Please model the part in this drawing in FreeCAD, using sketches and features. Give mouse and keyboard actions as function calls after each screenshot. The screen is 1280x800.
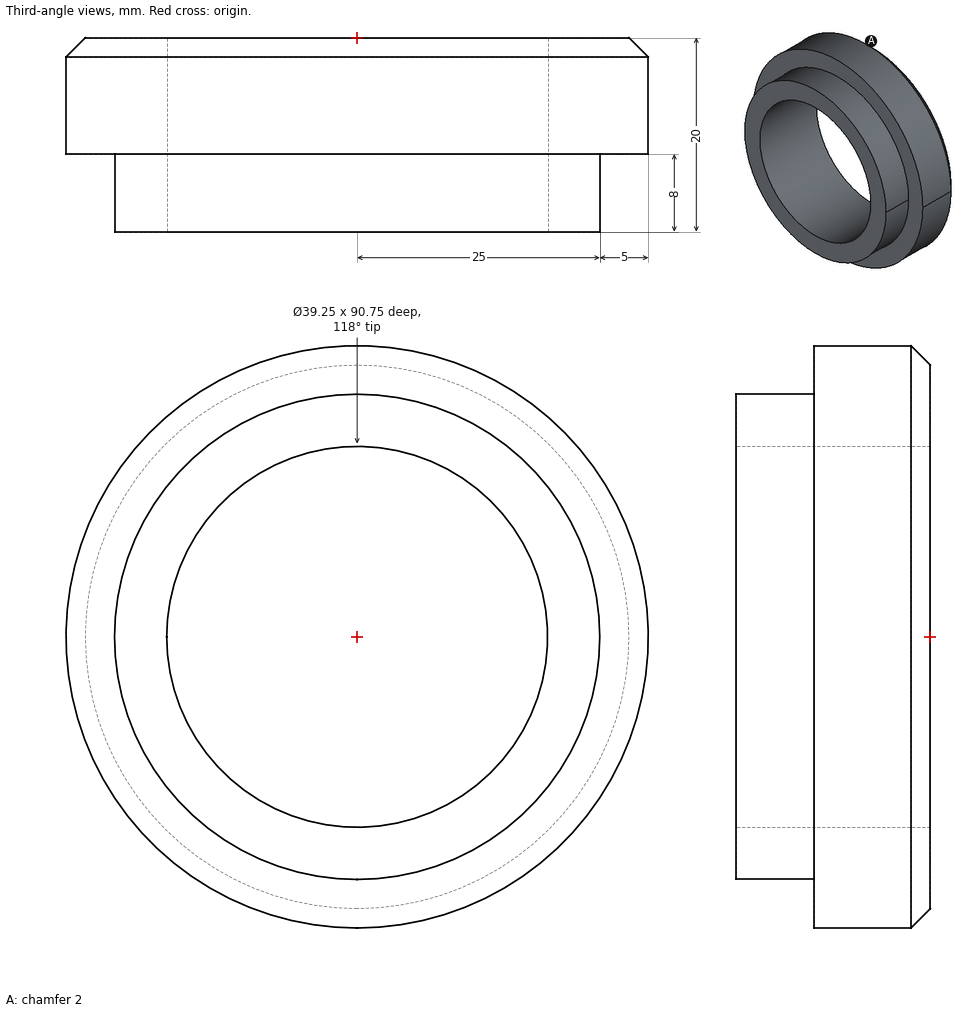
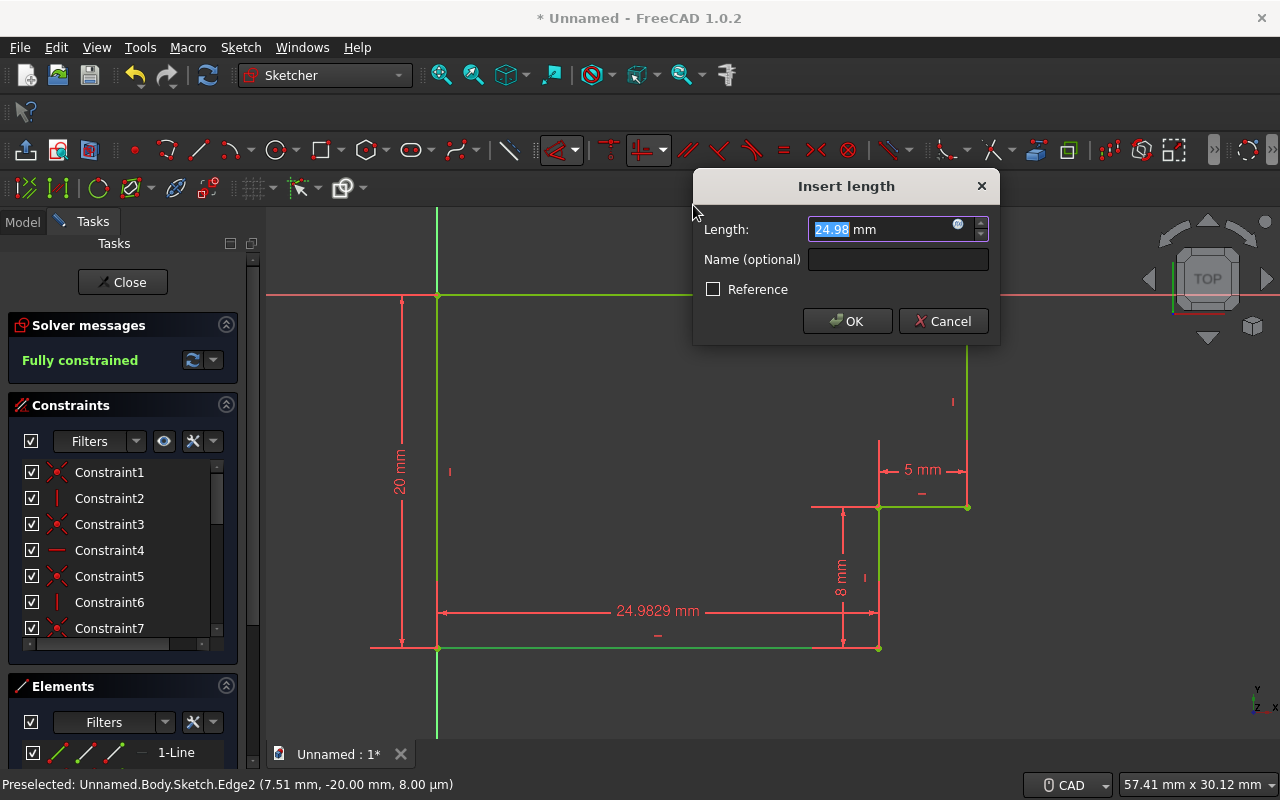
text(25)
key(Return)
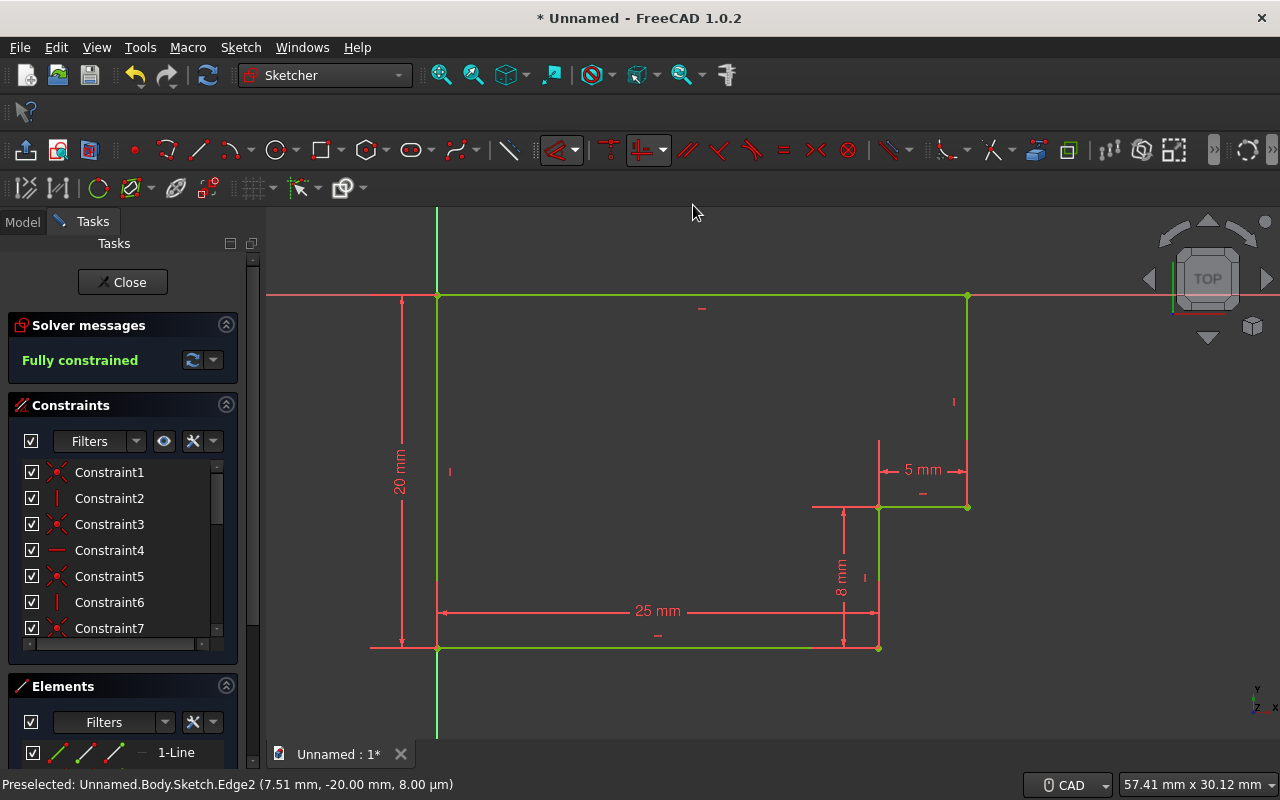
click(123, 282)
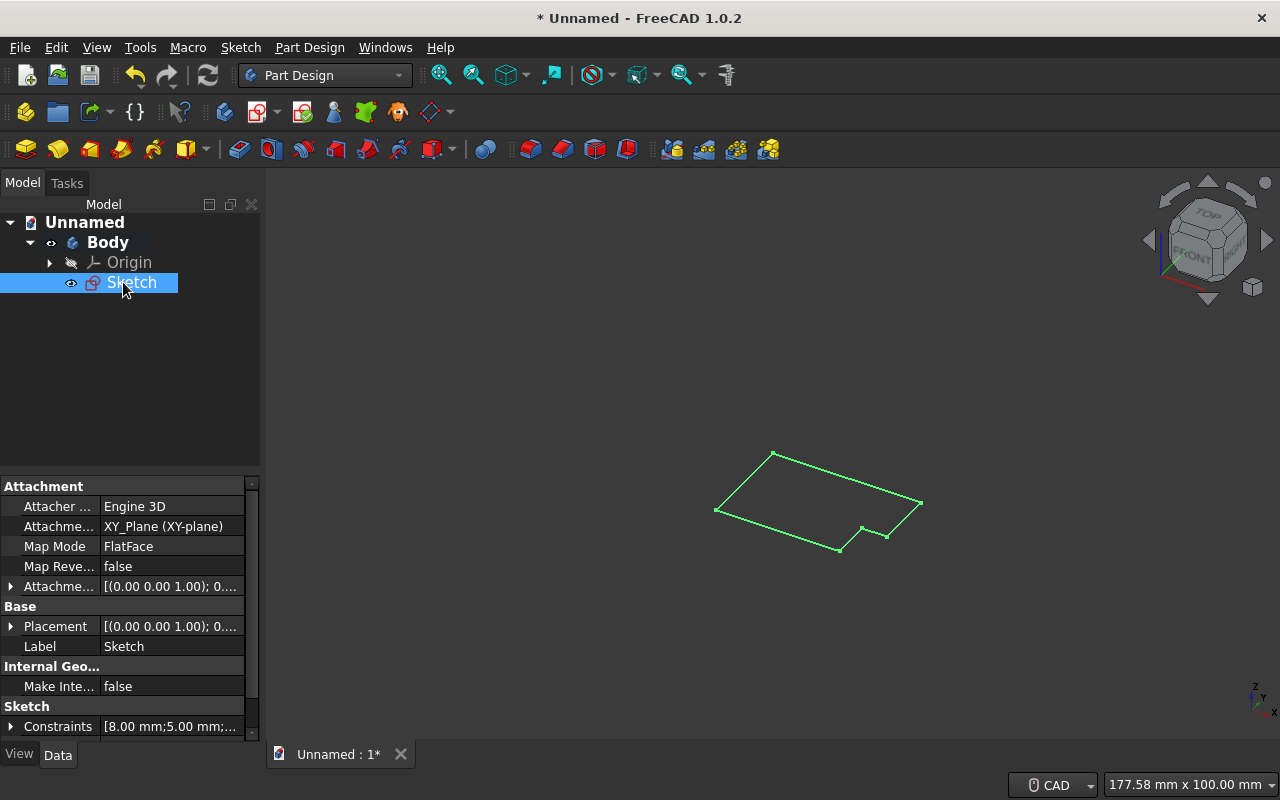
click(58, 150)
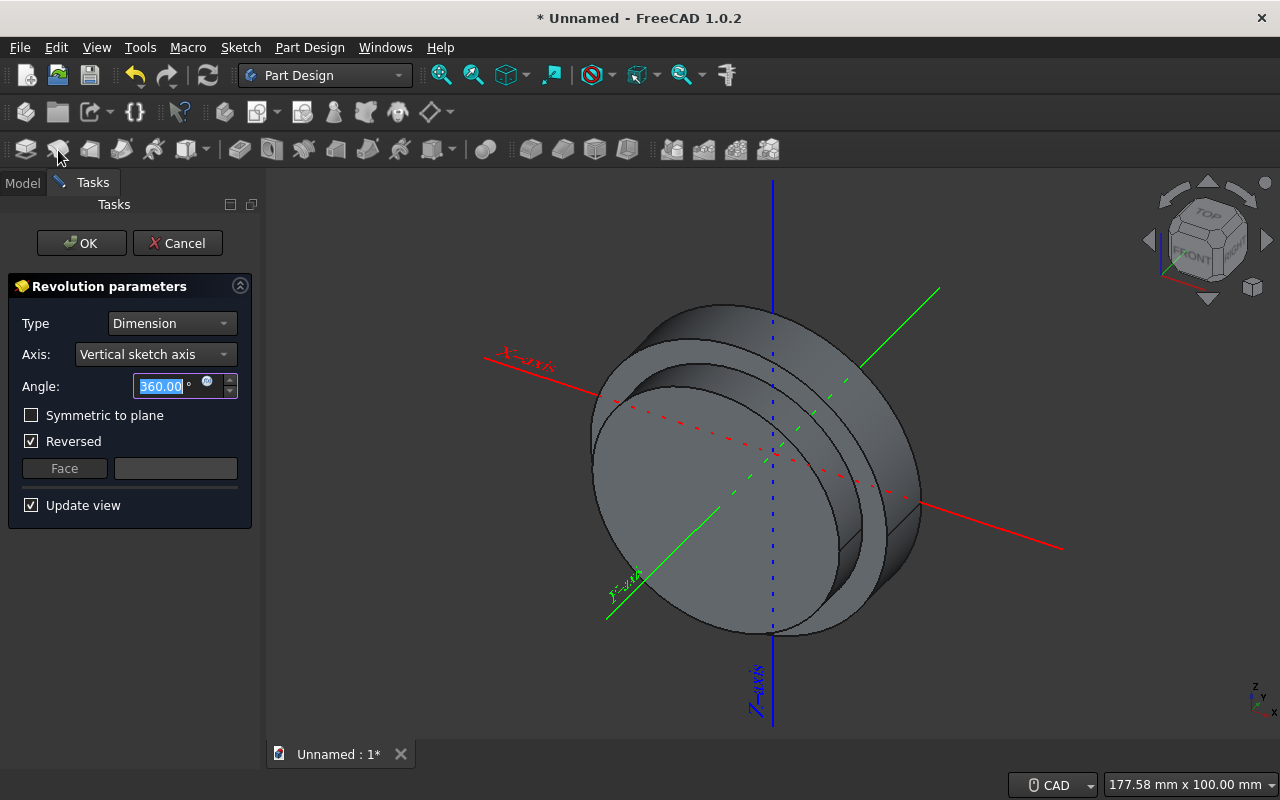
click(82, 243)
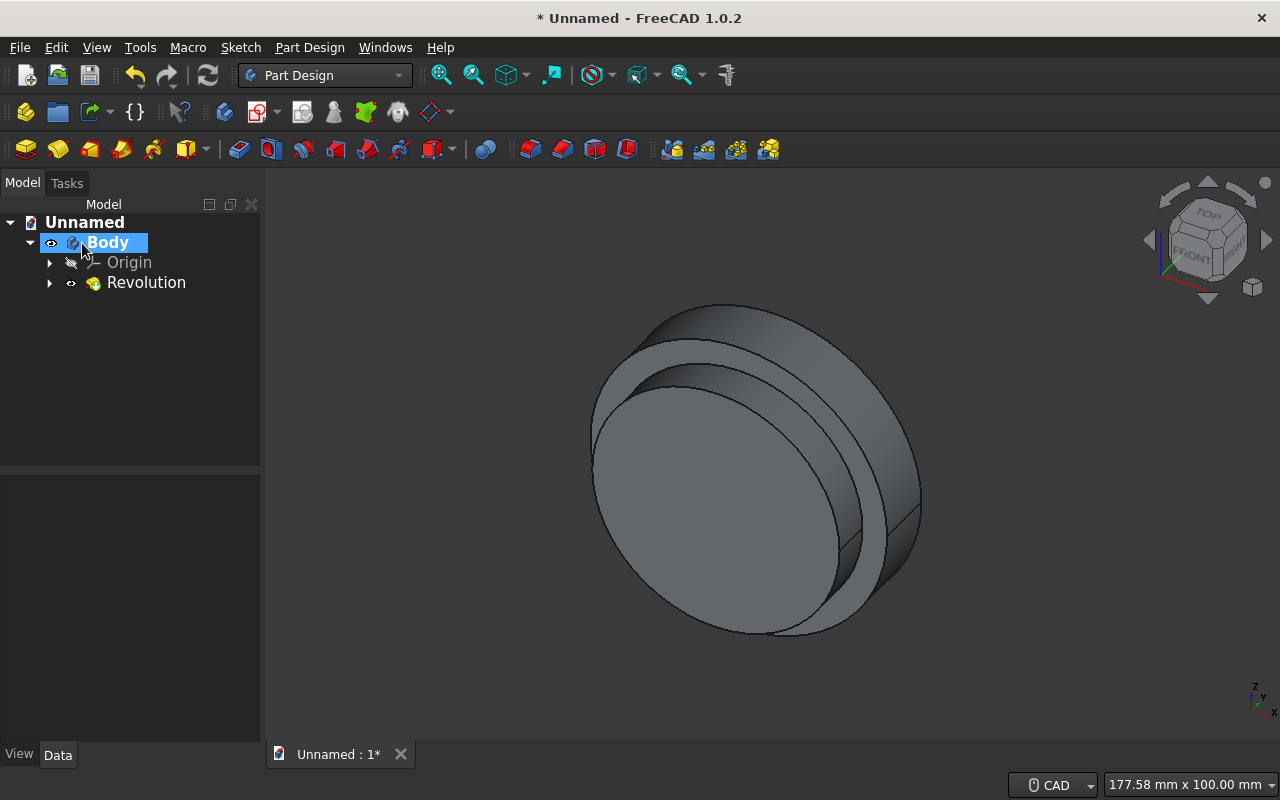
click(258, 112)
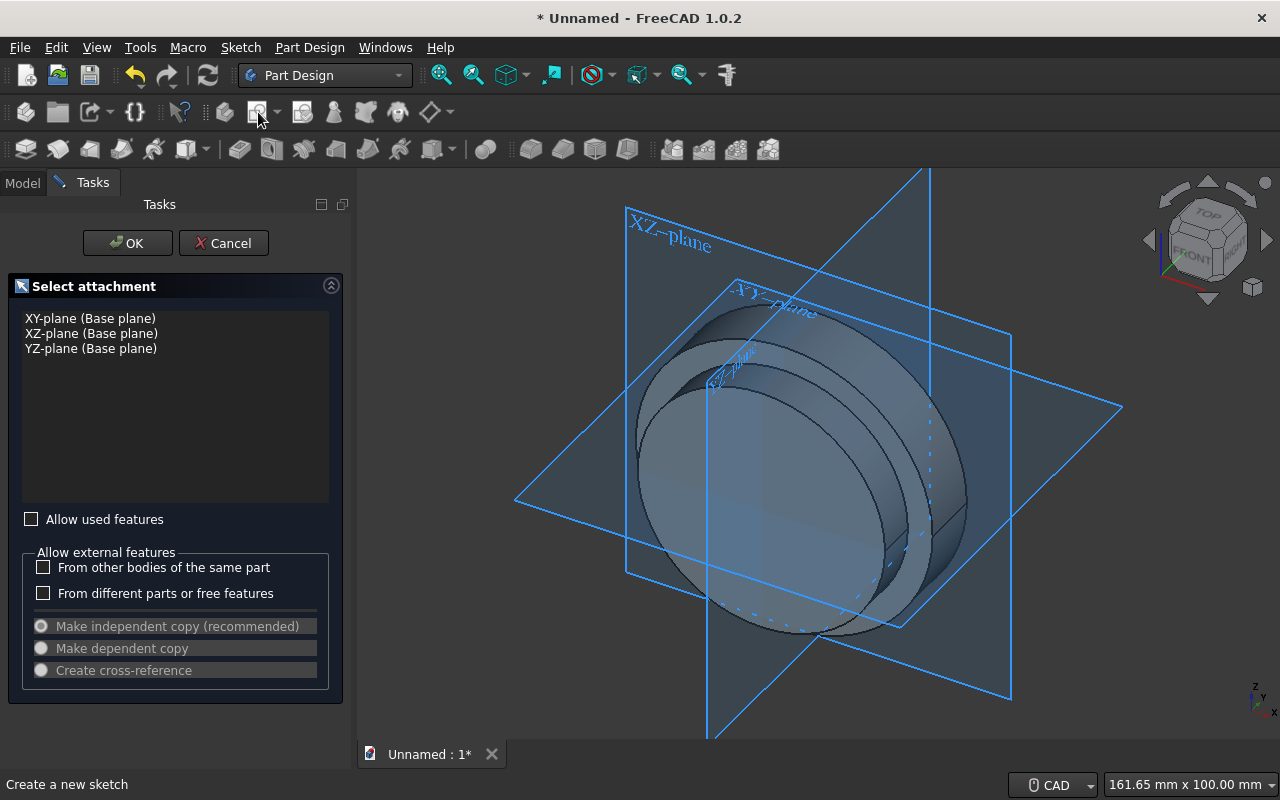
click(82, 334)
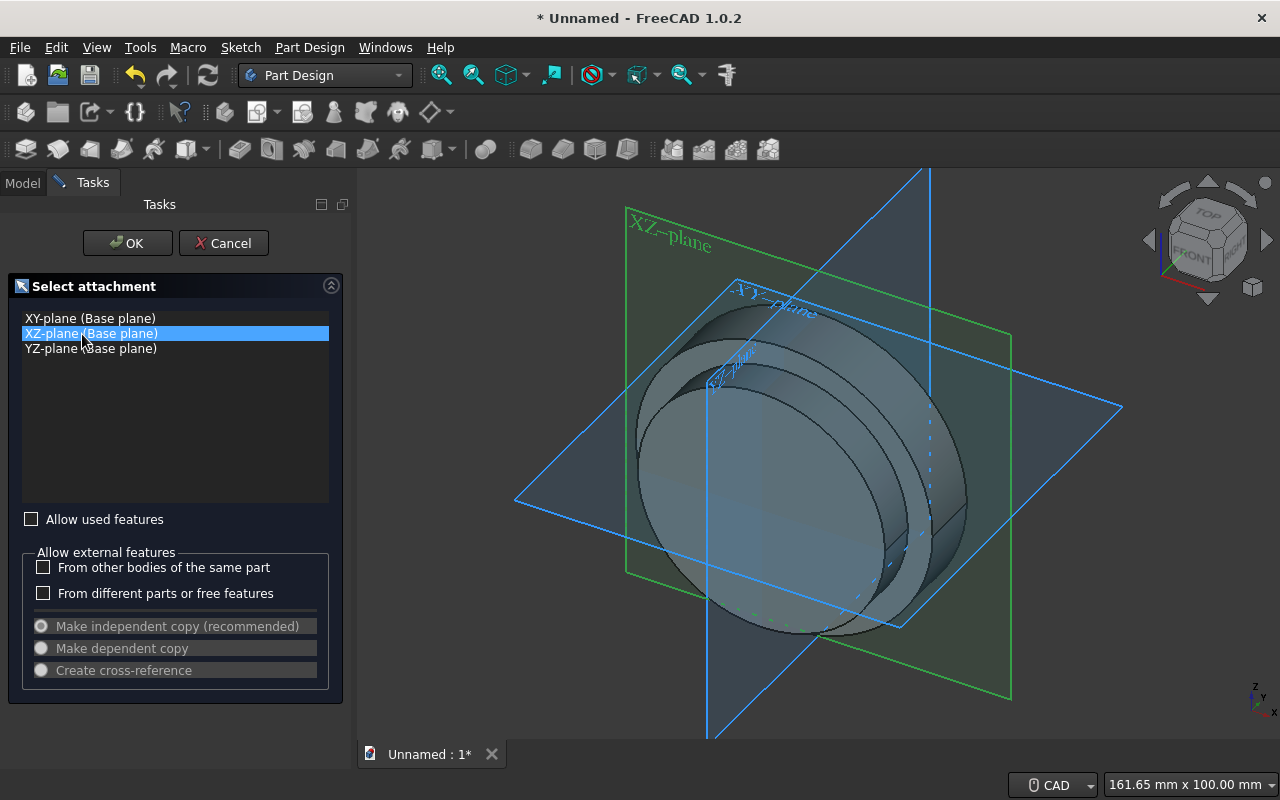
click(128, 243)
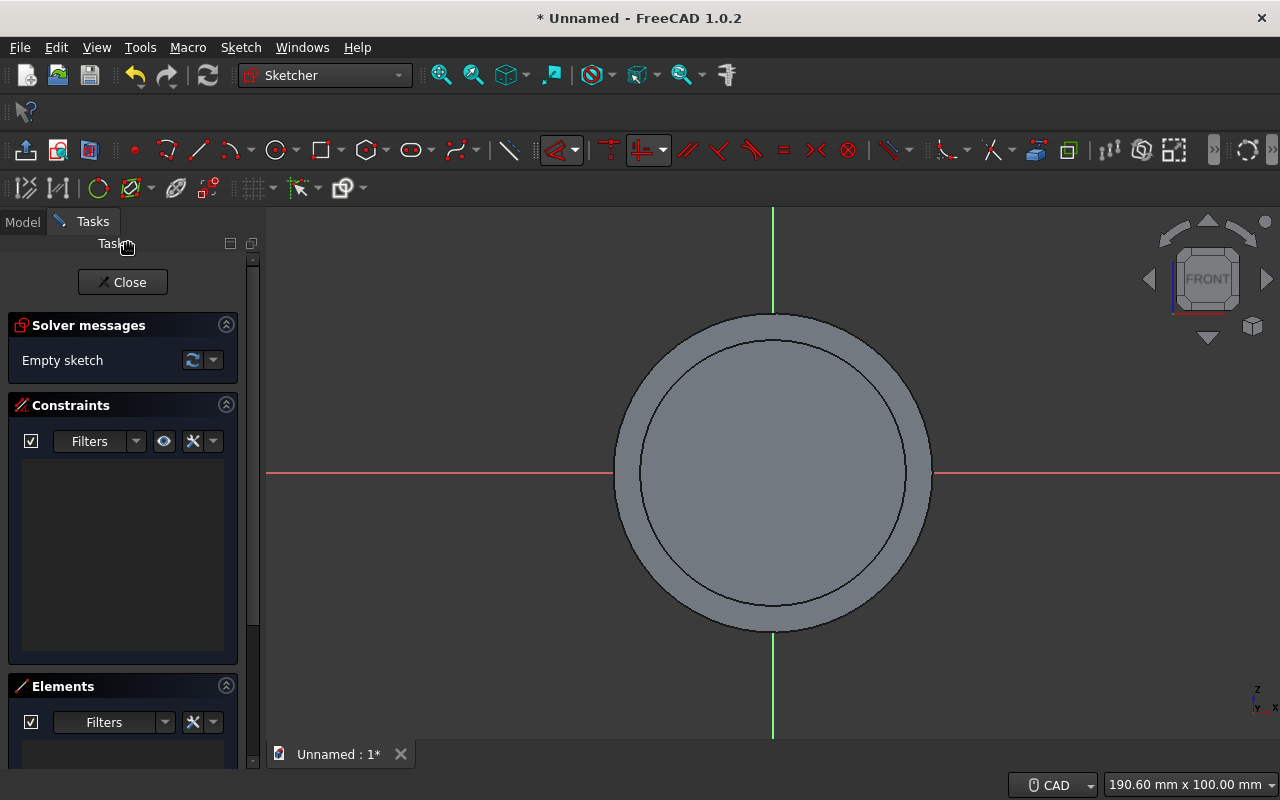
click(90, 150)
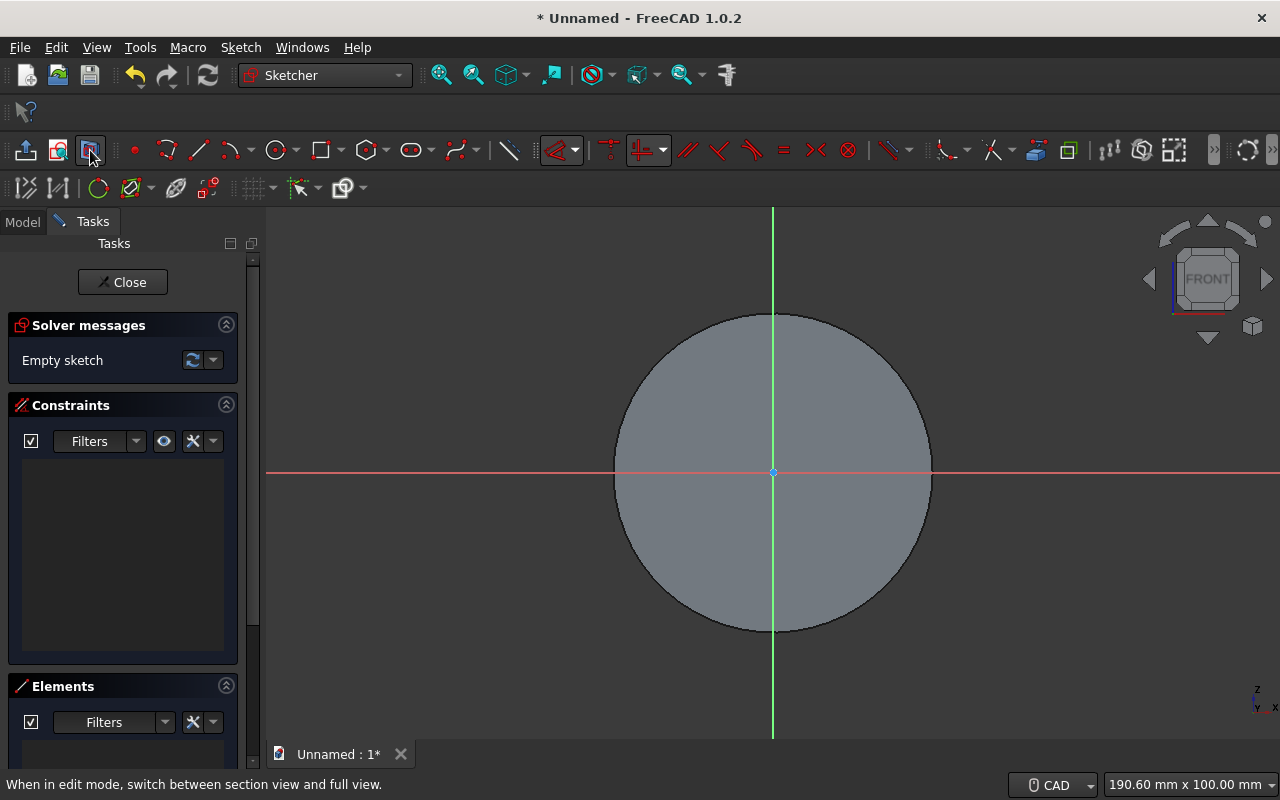
scroll(912, 473, up, 2)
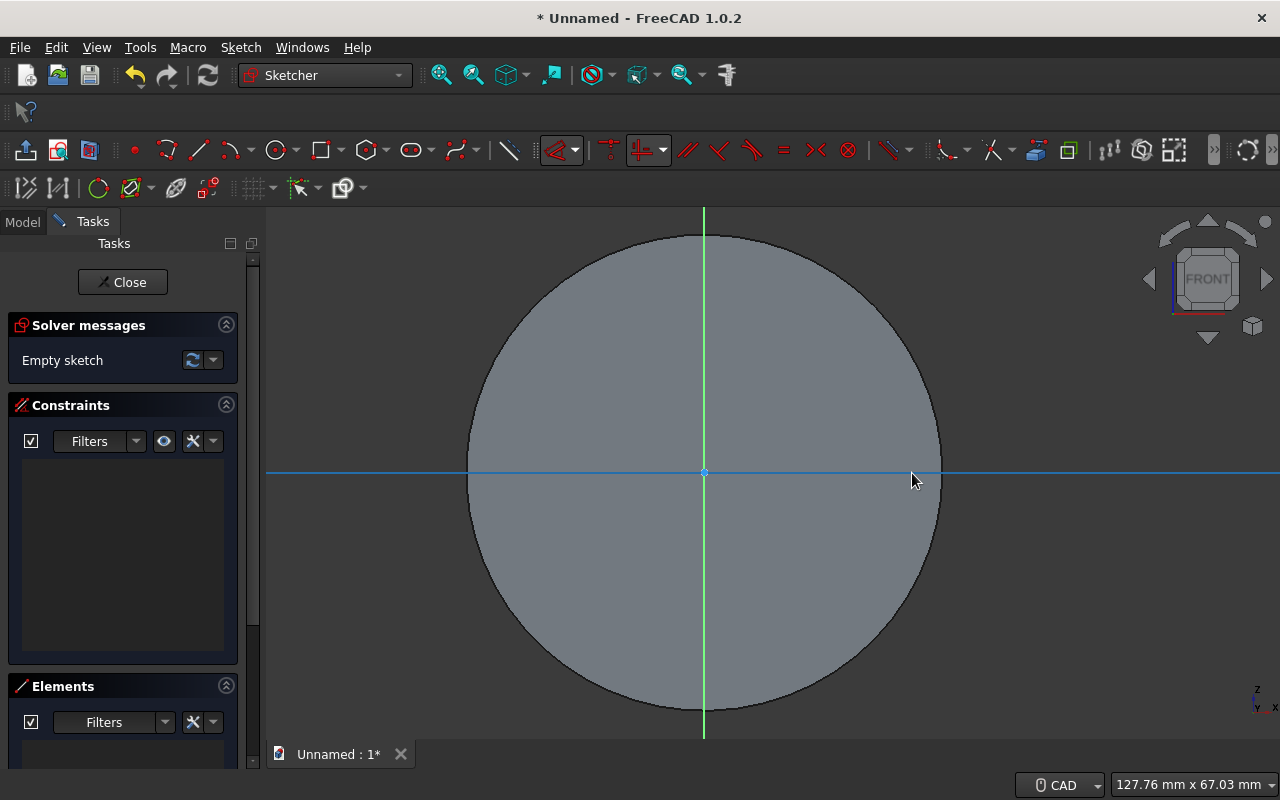
click(276, 150)